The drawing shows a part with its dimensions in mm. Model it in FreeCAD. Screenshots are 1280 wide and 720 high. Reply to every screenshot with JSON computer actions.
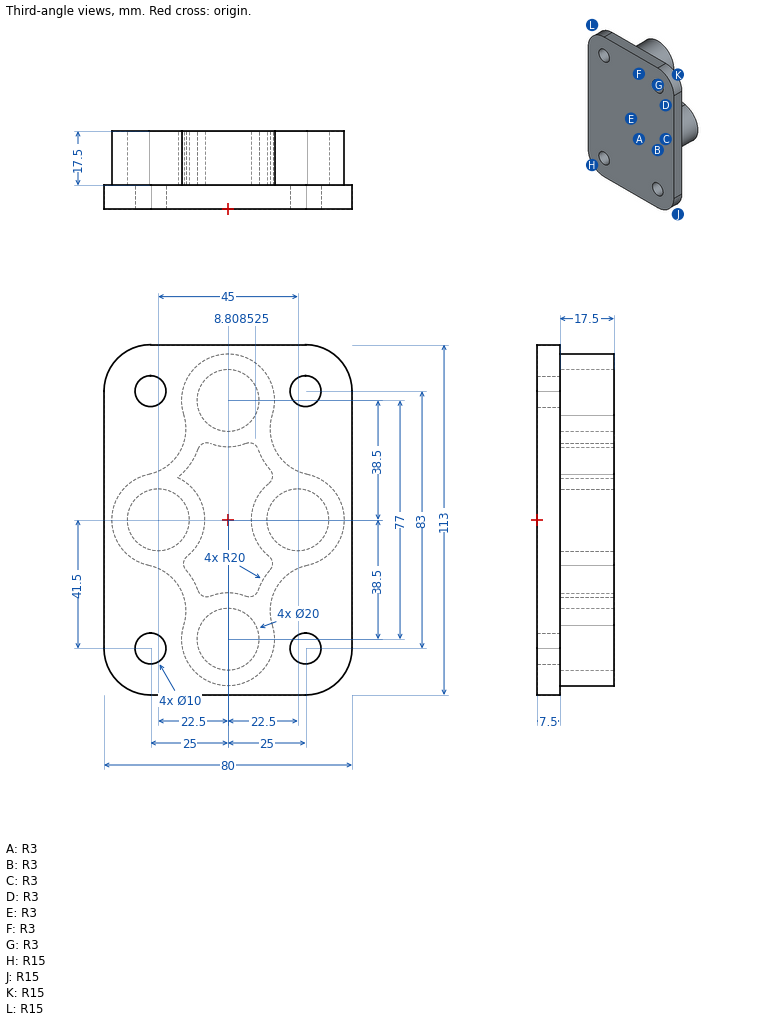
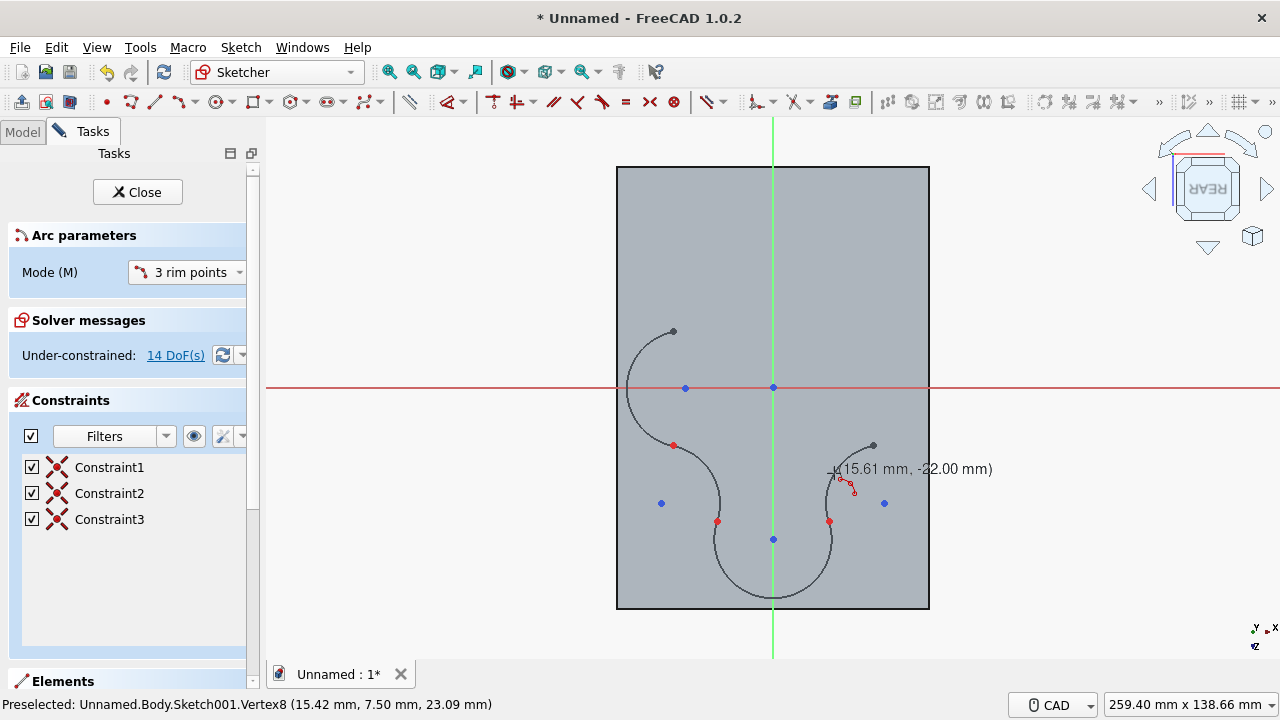
{"action": "left_click", "coordinate": [873, 446]}
{"action": "left_click", "coordinate": [873, 331]}
{"action": "left_click", "coordinate": [917, 404]}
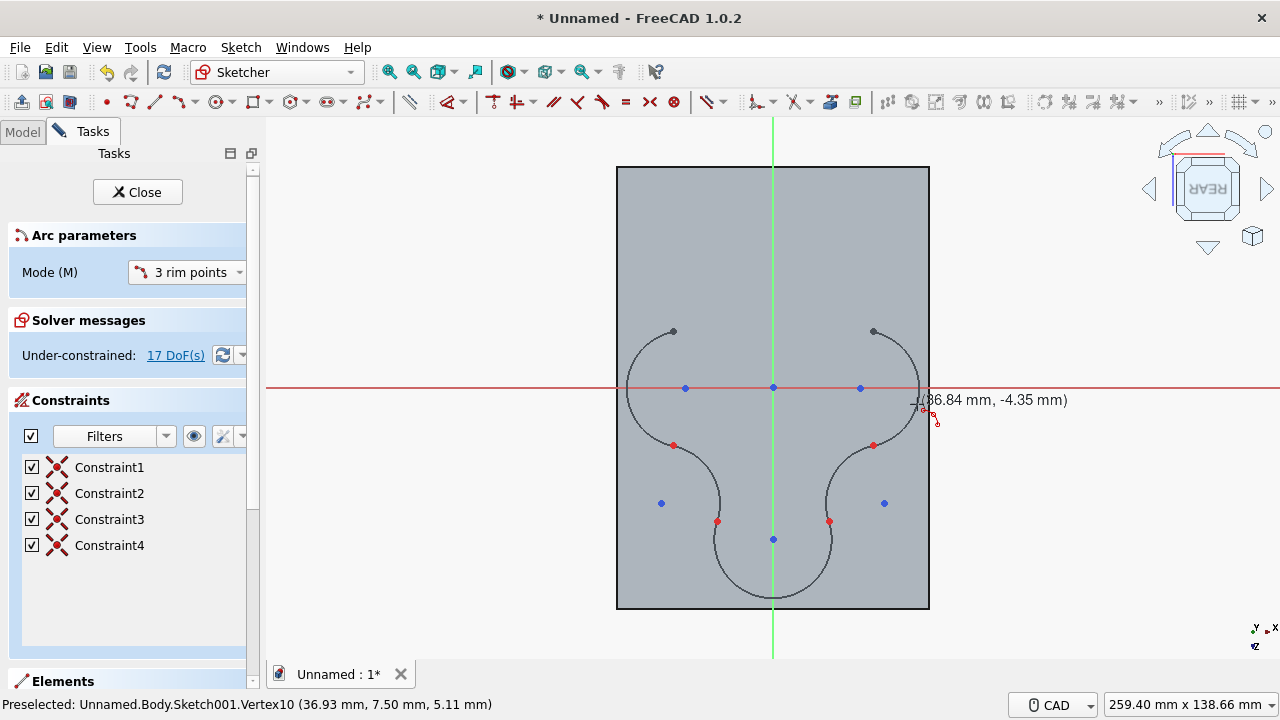
{"action": "left_click", "coordinate": [873, 332]}
{"action": "left_click", "coordinate": [829, 255]}
{"action": "left_click", "coordinate": [834, 303]}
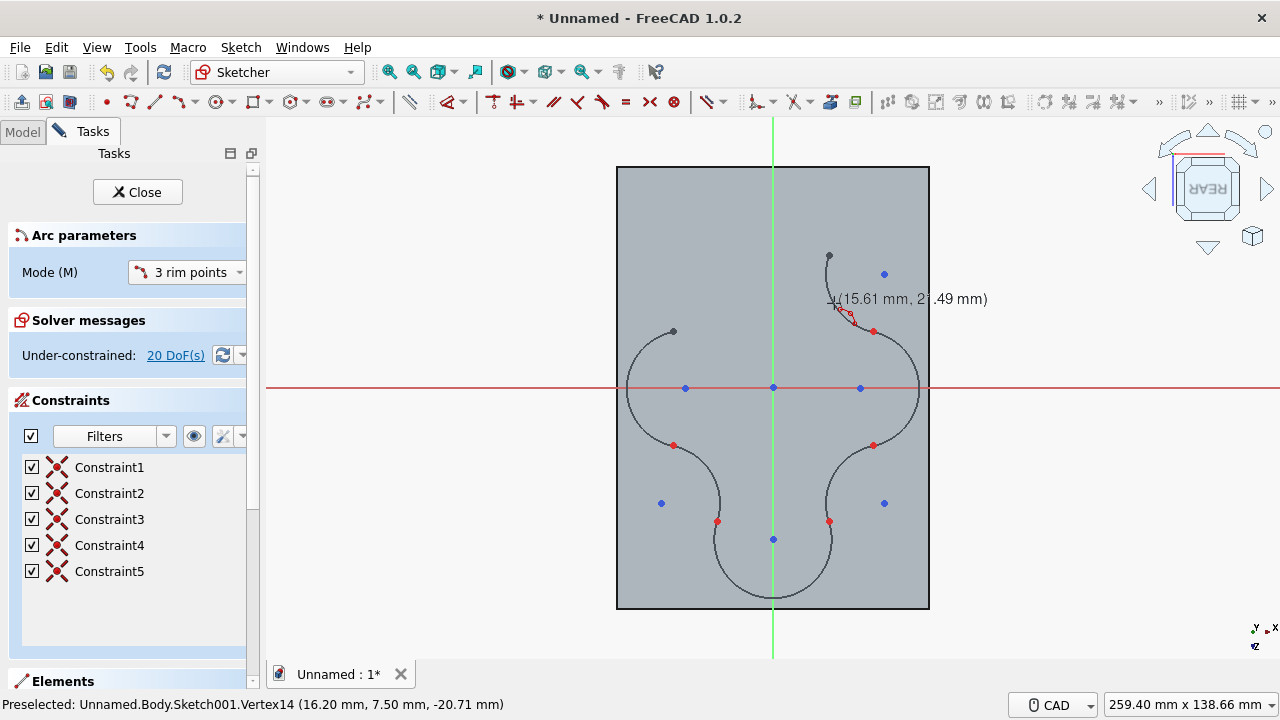
{"action": "left_click", "coordinate": [829, 256]}
{"action": "left_click", "coordinate": [717, 255]}
{"action": "left_click", "coordinate": [795, 183]}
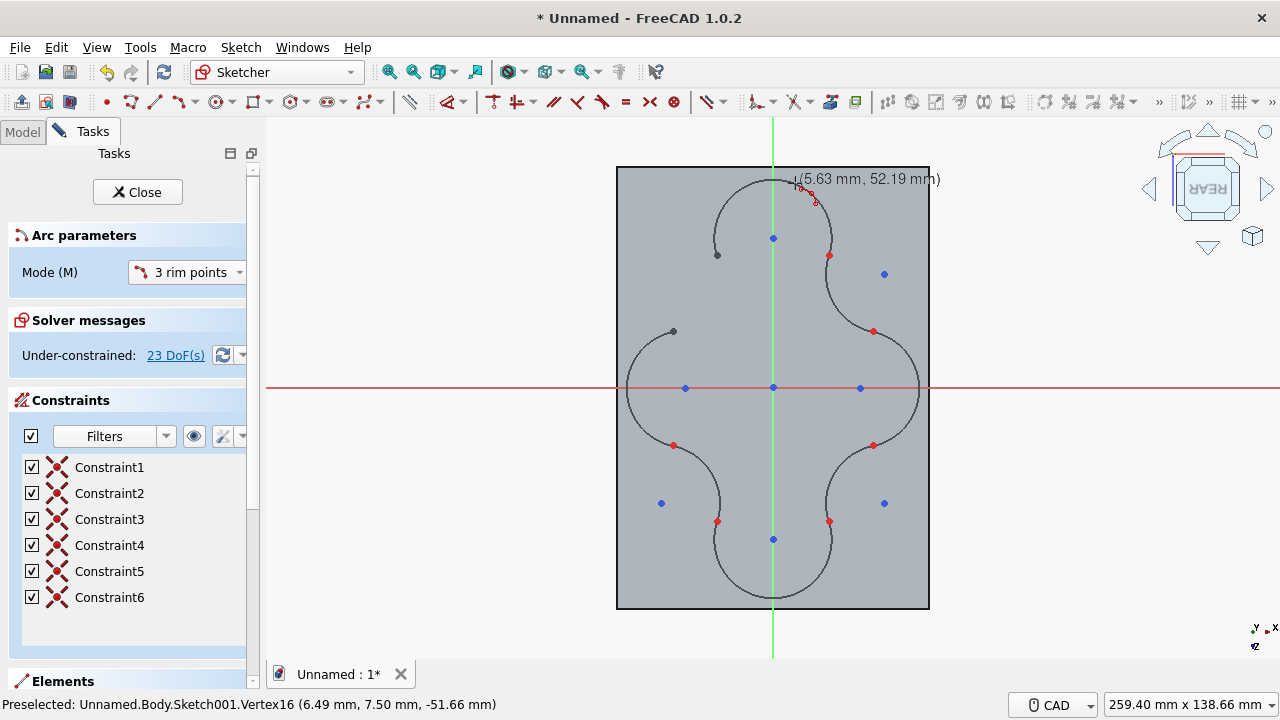
{"action": "left_click", "coordinate": [717, 256]}
{"action": "left_click", "coordinate": [673, 332]}
{"action": "left_click", "coordinate": [712, 303]}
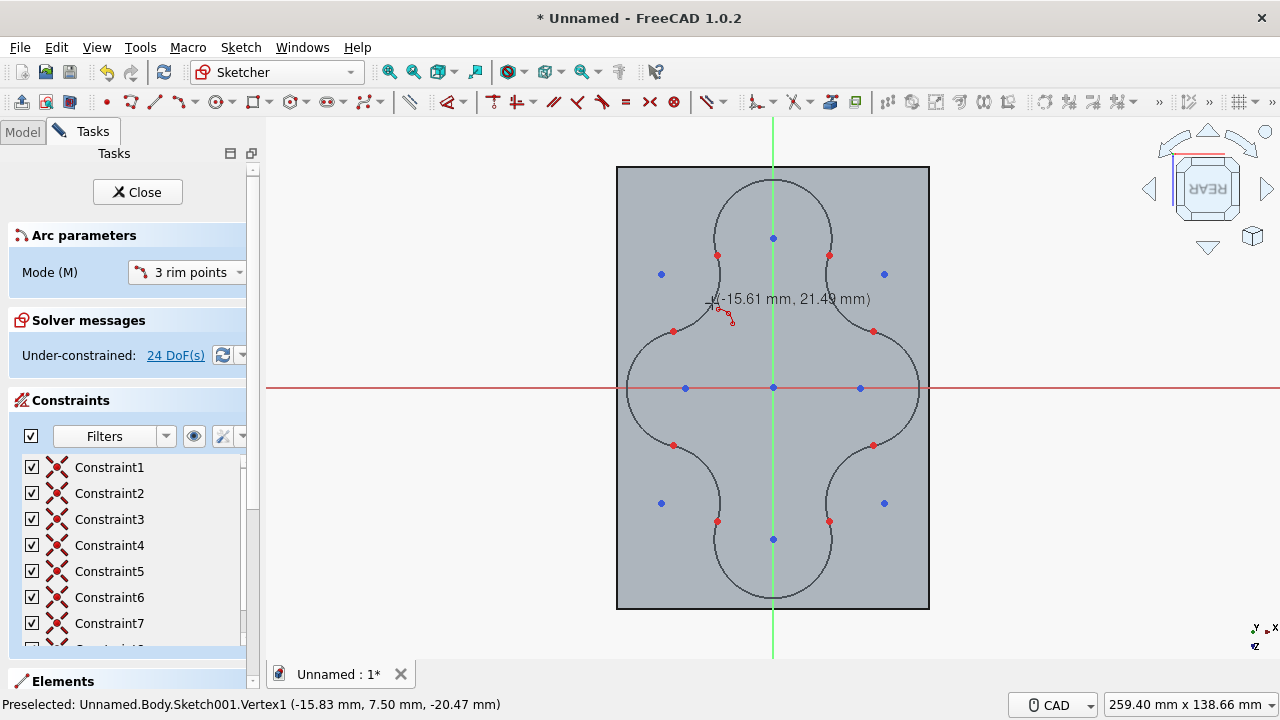
{"action": "left_click", "coordinate": [837, 335]}
{"action": "left_click", "coordinate": [837, 441]}
{"action": "left_click", "coordinate": [808, 362]}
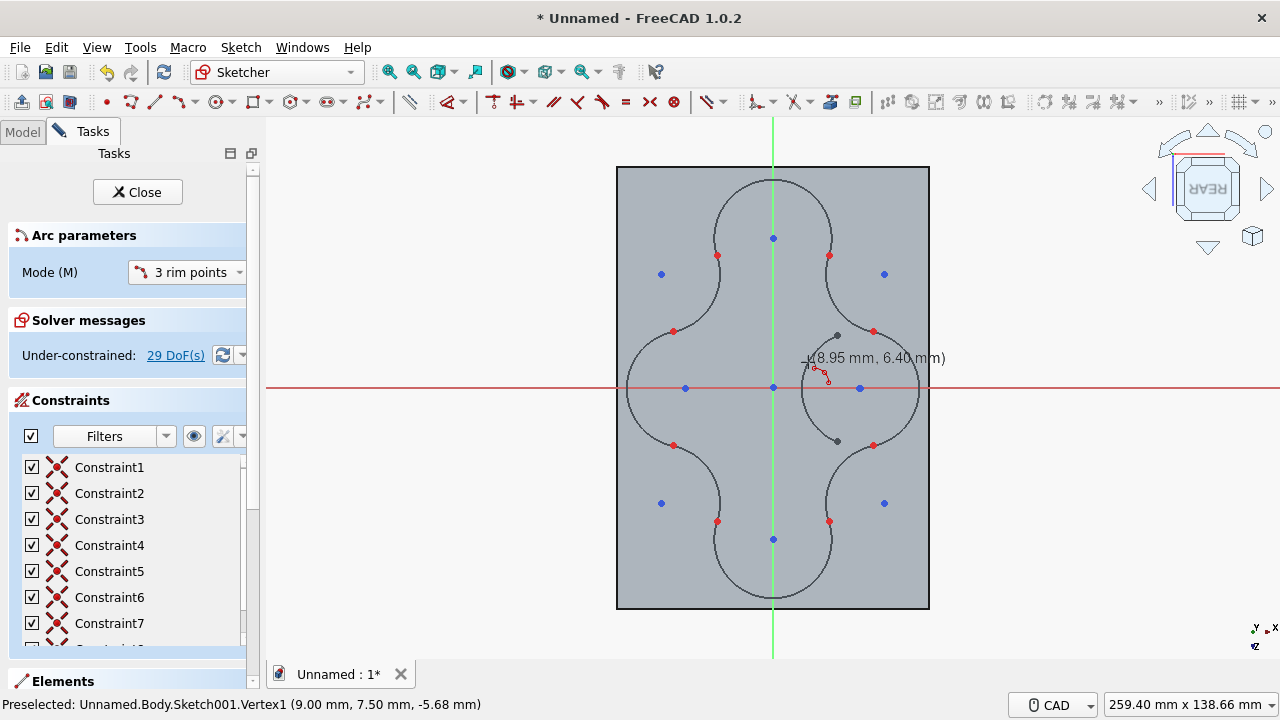
{"action": "left_click", "coordinate": [837, 442]}
{"action": "left_click", "coordinate": [807, 491]}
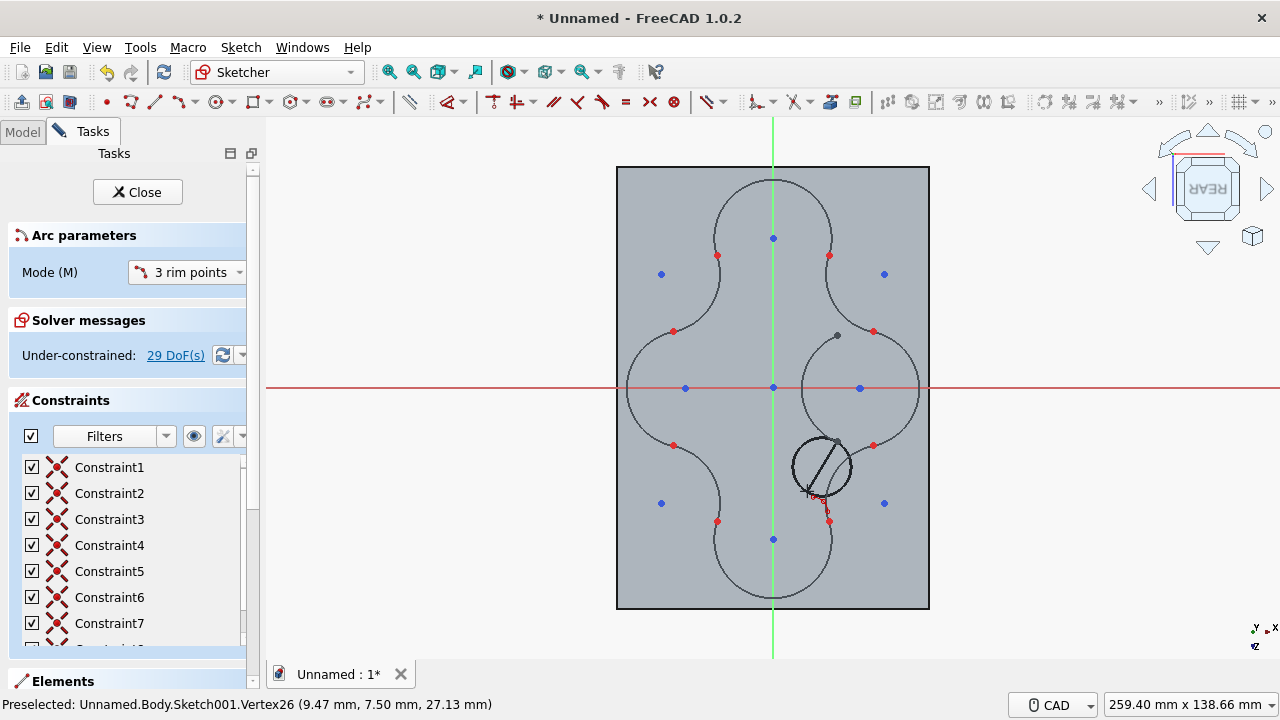
{"action": "scroll", "coordinate": [817, 463], "scroll_direction": "up", "scroll_amount": 6}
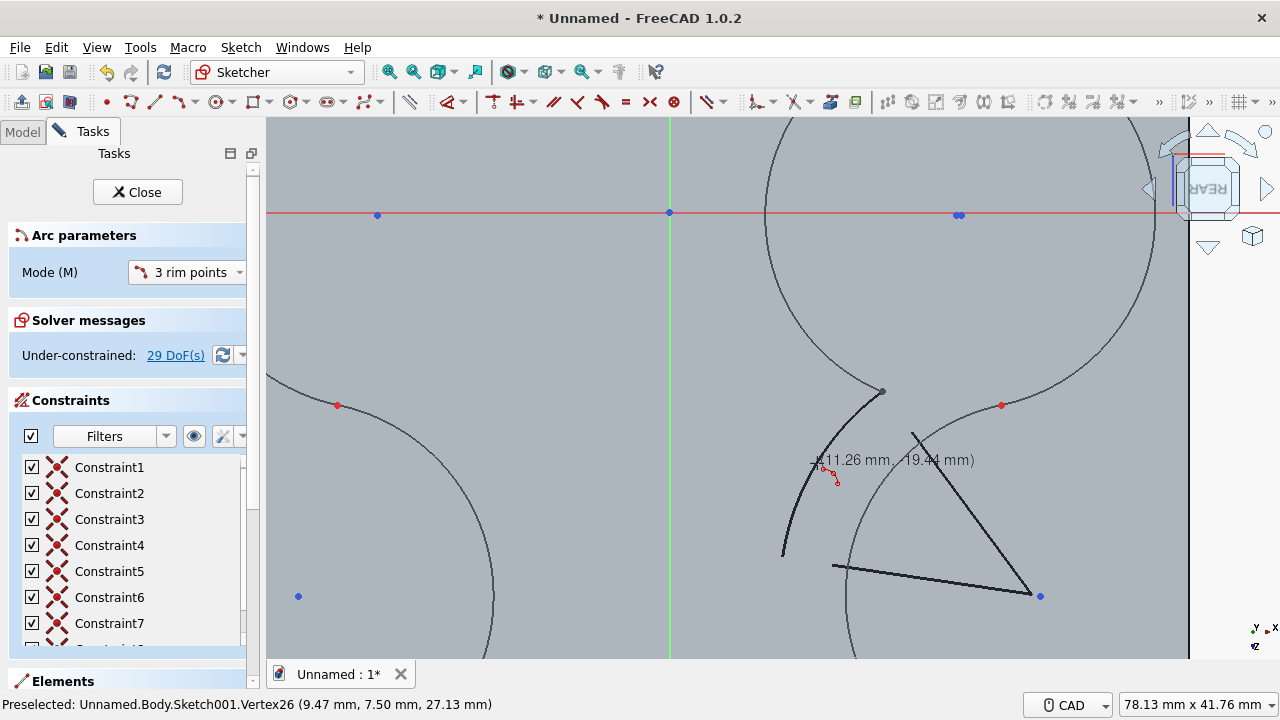
{"action": "left_click", "coordinate": [816, 463]}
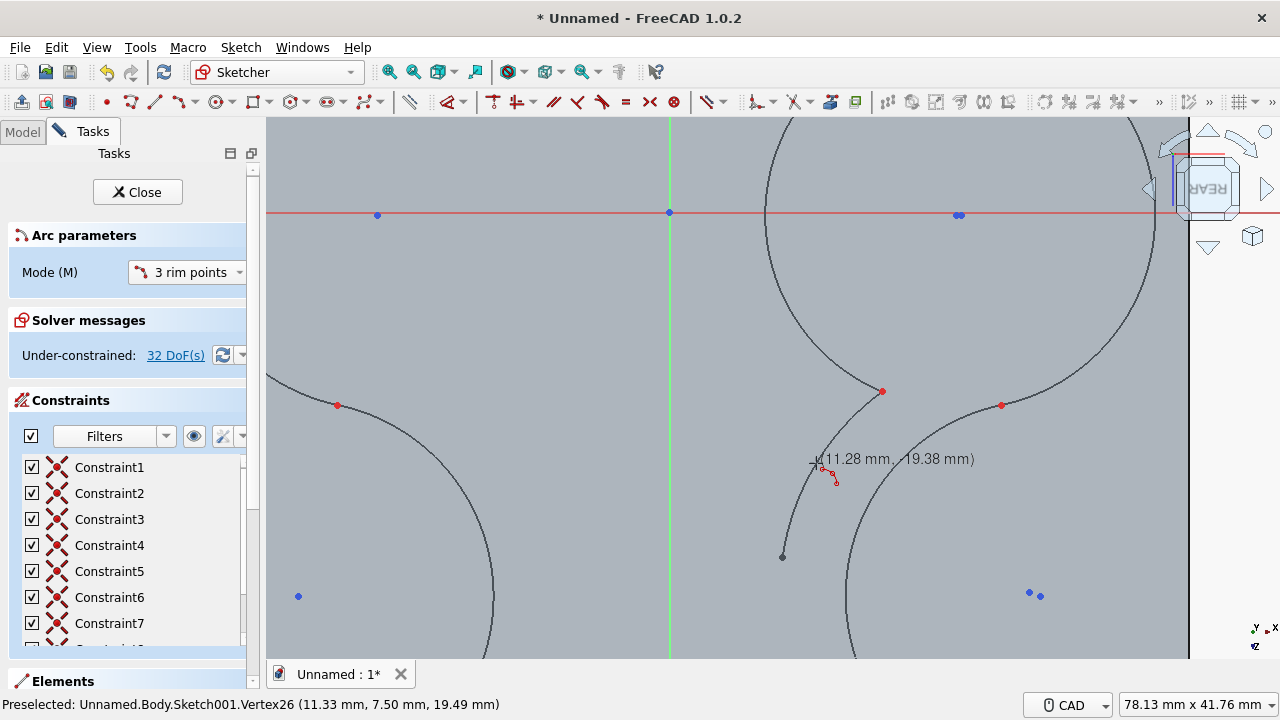
{"action": "left_click", "coordinate": [783, 558]}
{"action": "left_click", "coordinate": [555, 555]}
{"action": "left_click", "coordinate": [718, 524]}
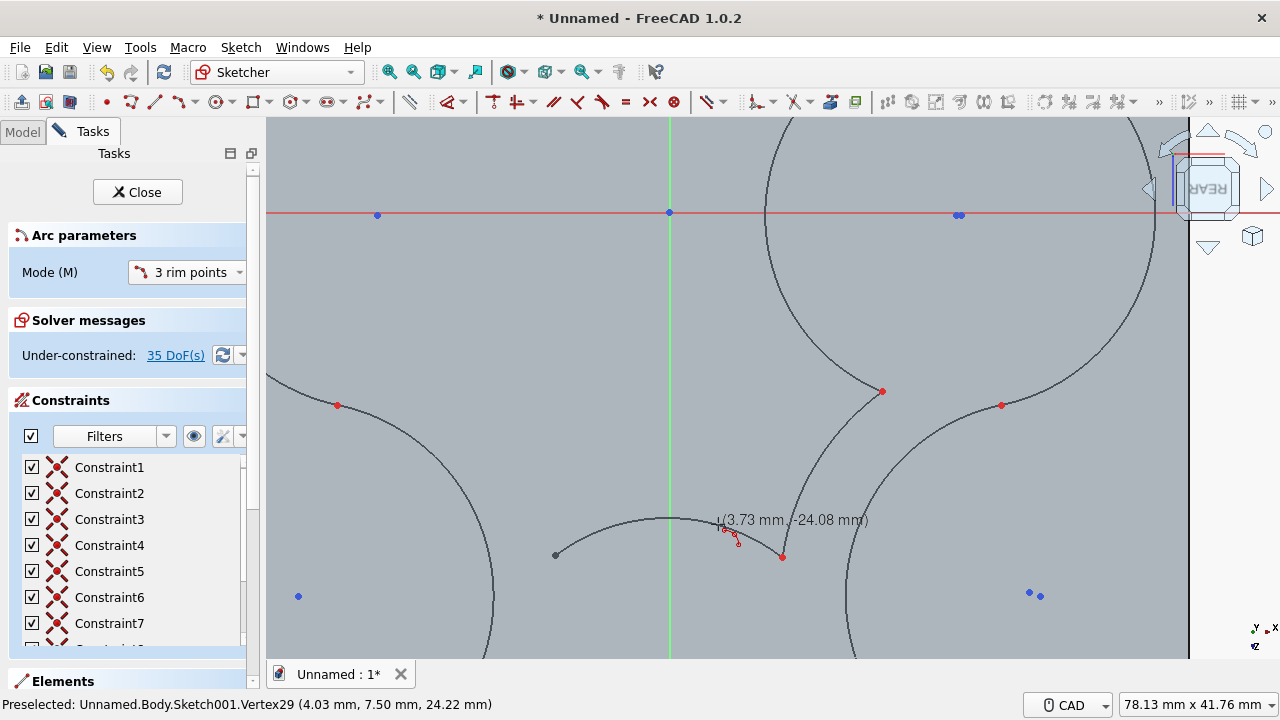
{"action": "left_click", "coordinate": [555, 556]}
{"action": "left_click", "coordinate": [459, 389]}
{"action": "left_click", "coordinate": [523, 463]}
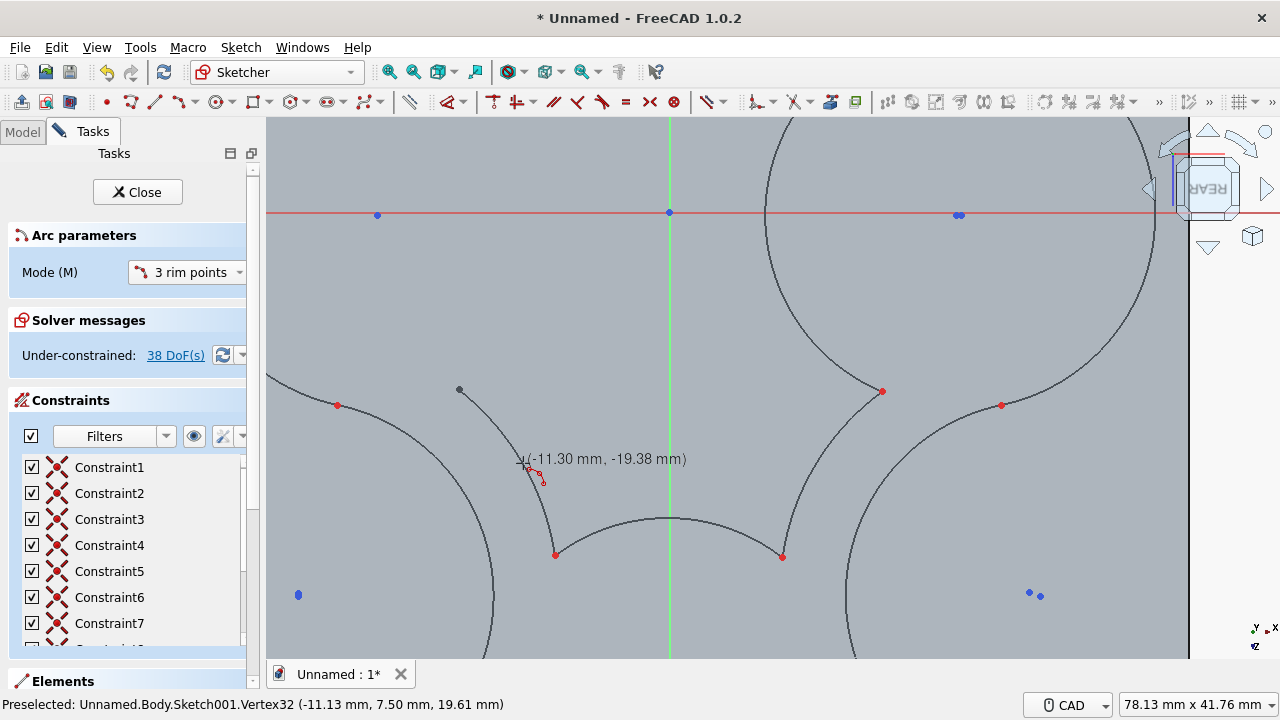
{"action": "left_click", "coordinate": [459, 390]}